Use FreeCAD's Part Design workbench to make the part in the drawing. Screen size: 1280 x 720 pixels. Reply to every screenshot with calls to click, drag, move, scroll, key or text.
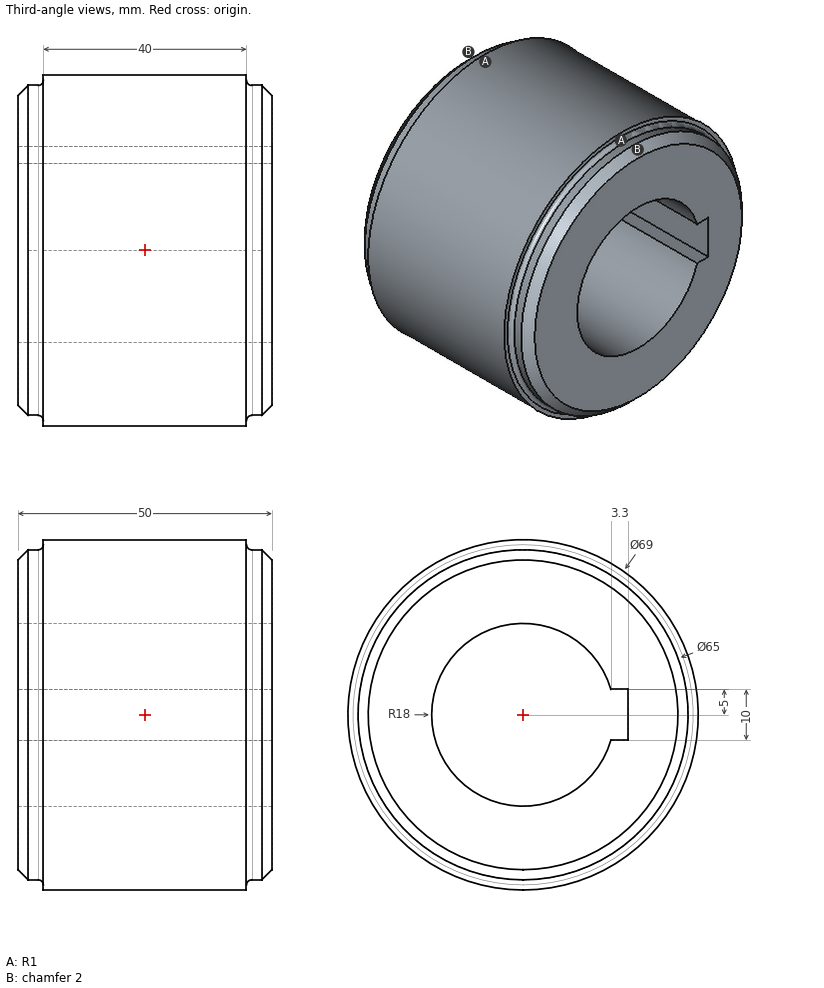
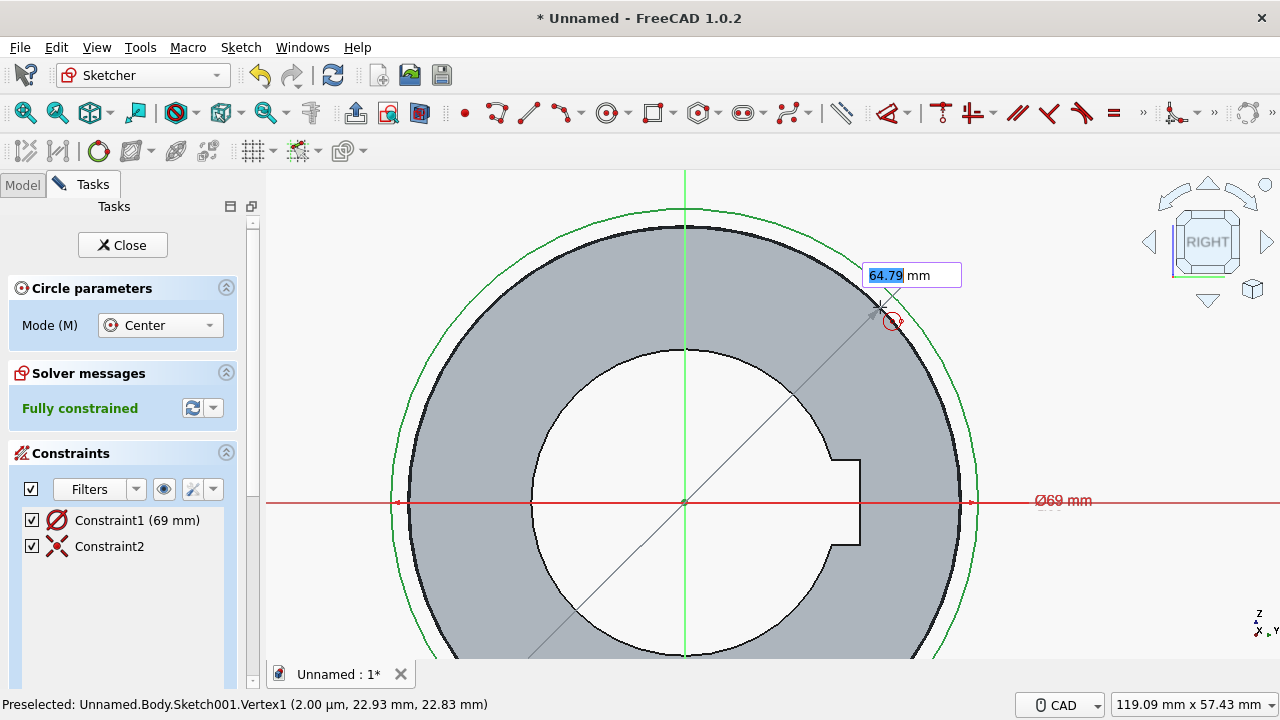
text(65)
key(Return)
key(Escape)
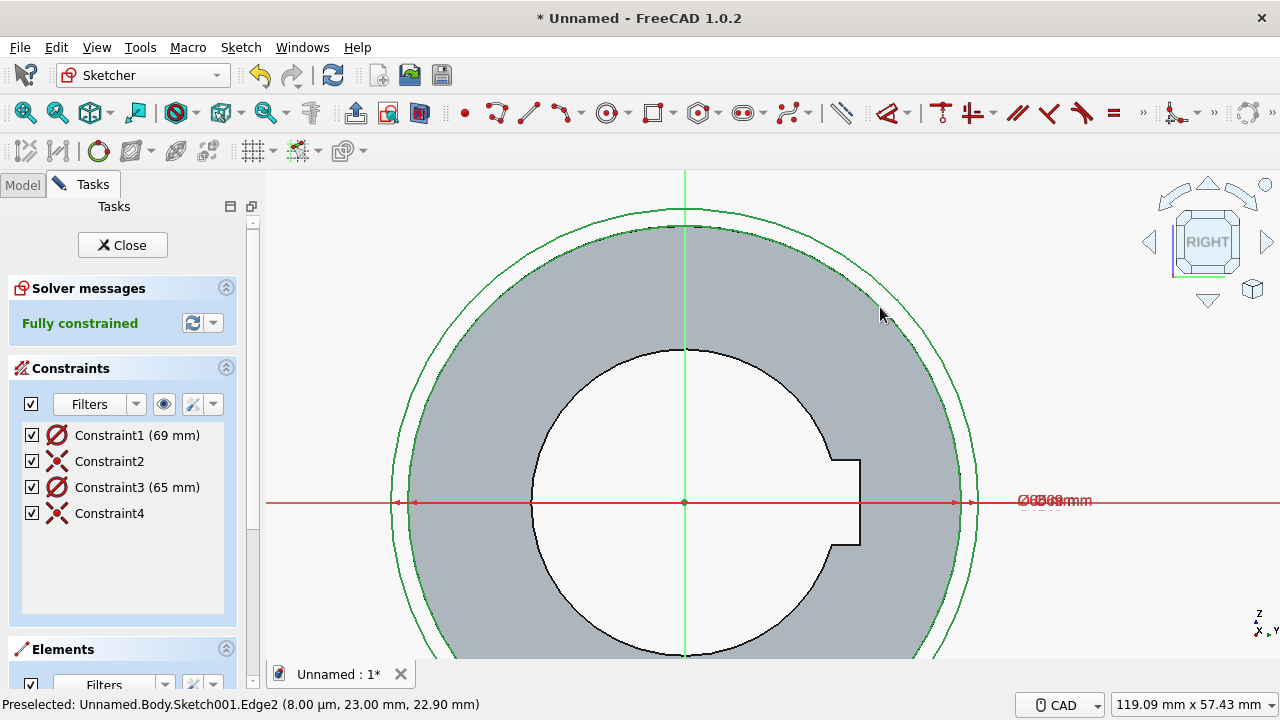
click(123, 245)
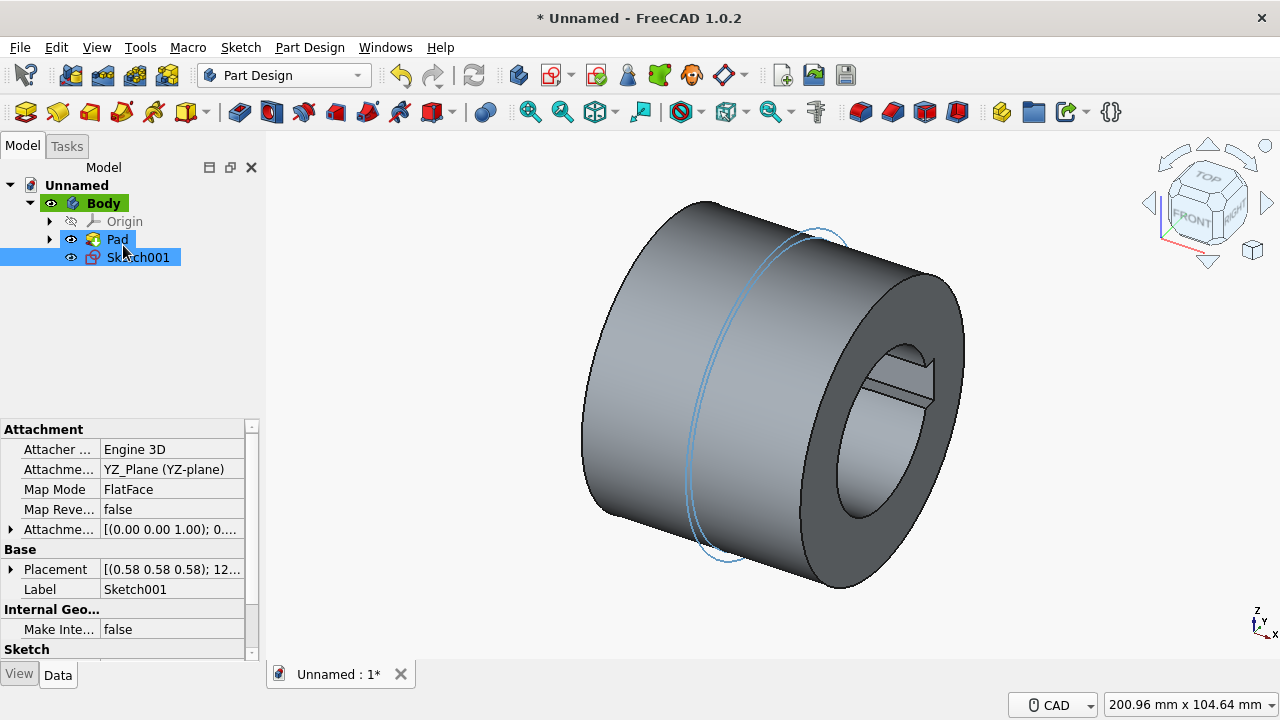
click(26, 112)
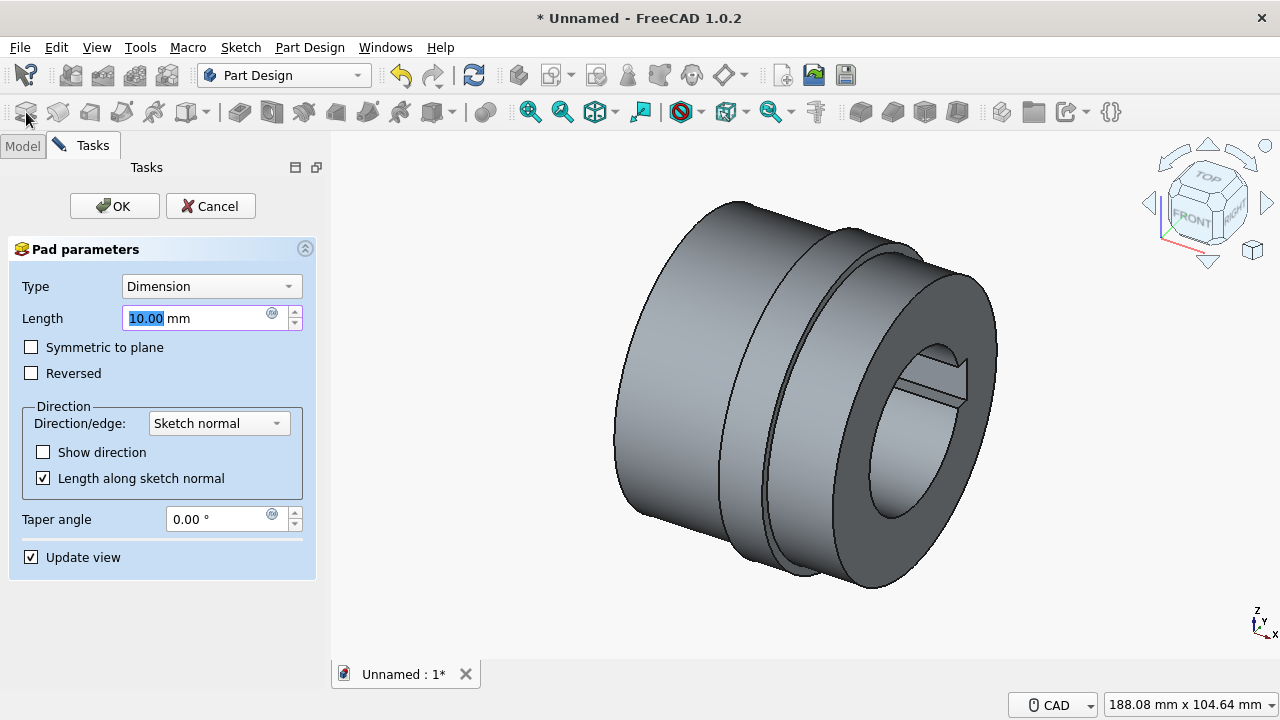
text(40)
key(Tab)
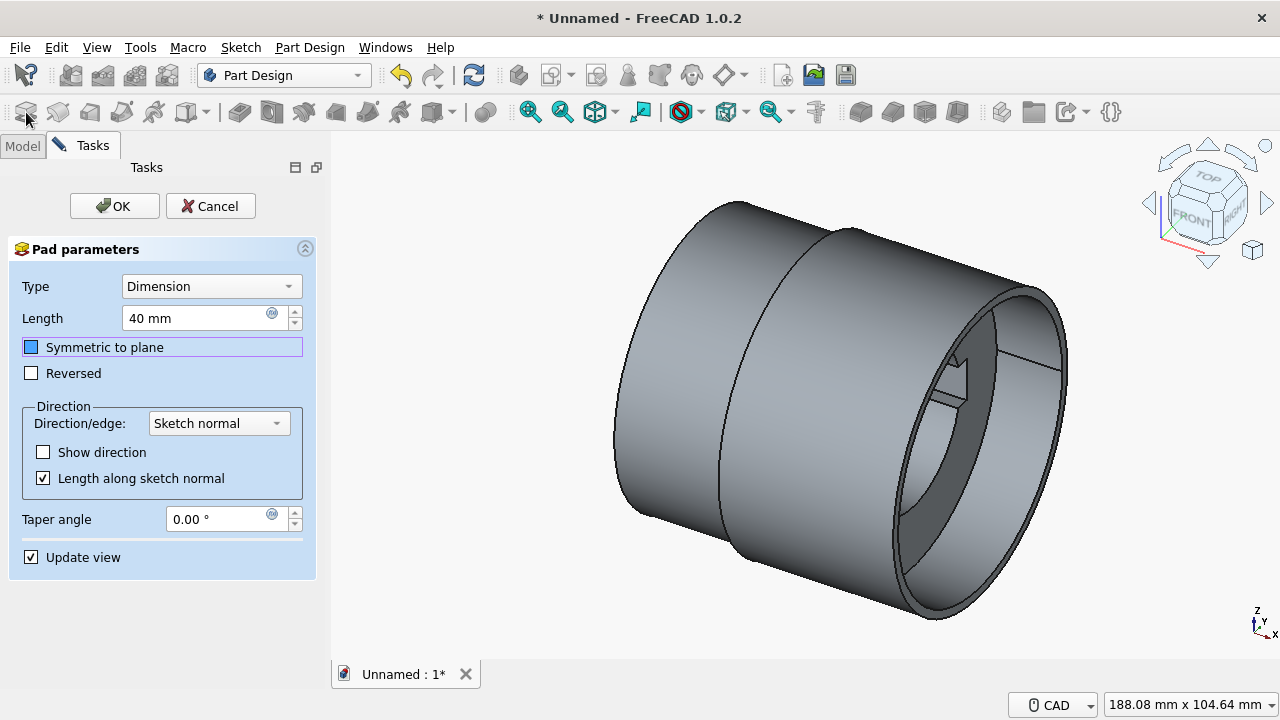
click(30, 347)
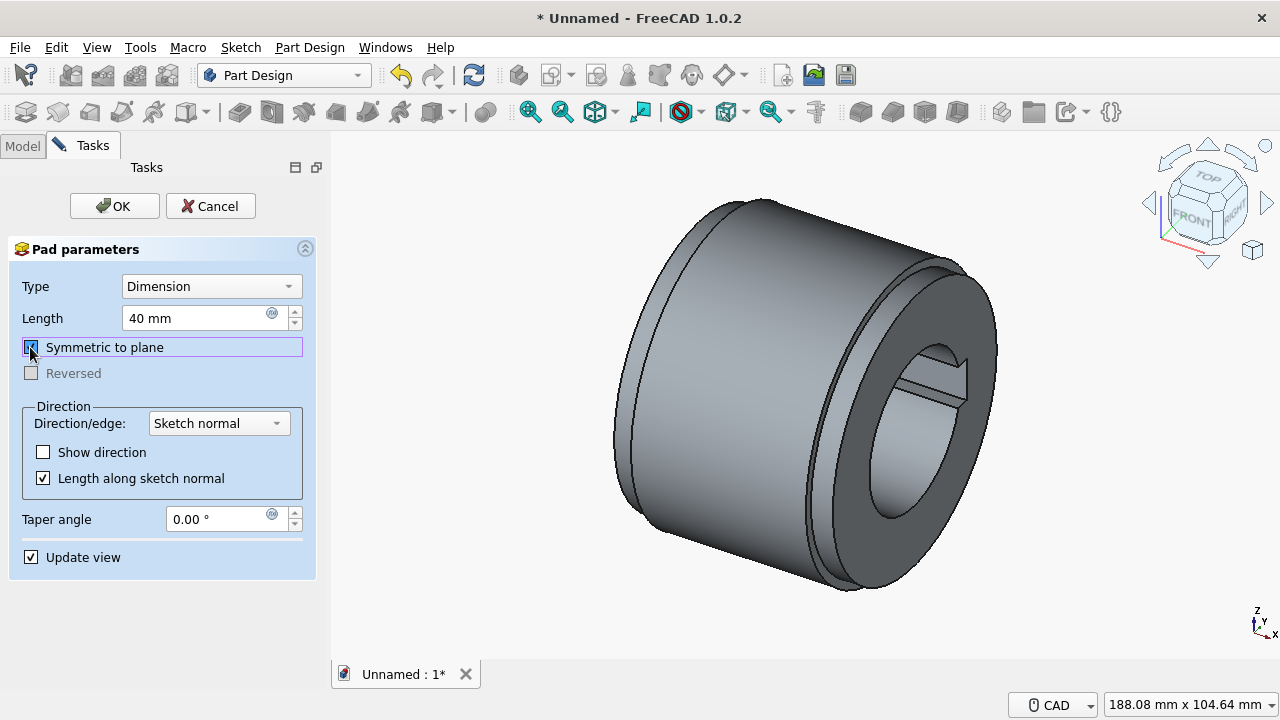
click(115, 206)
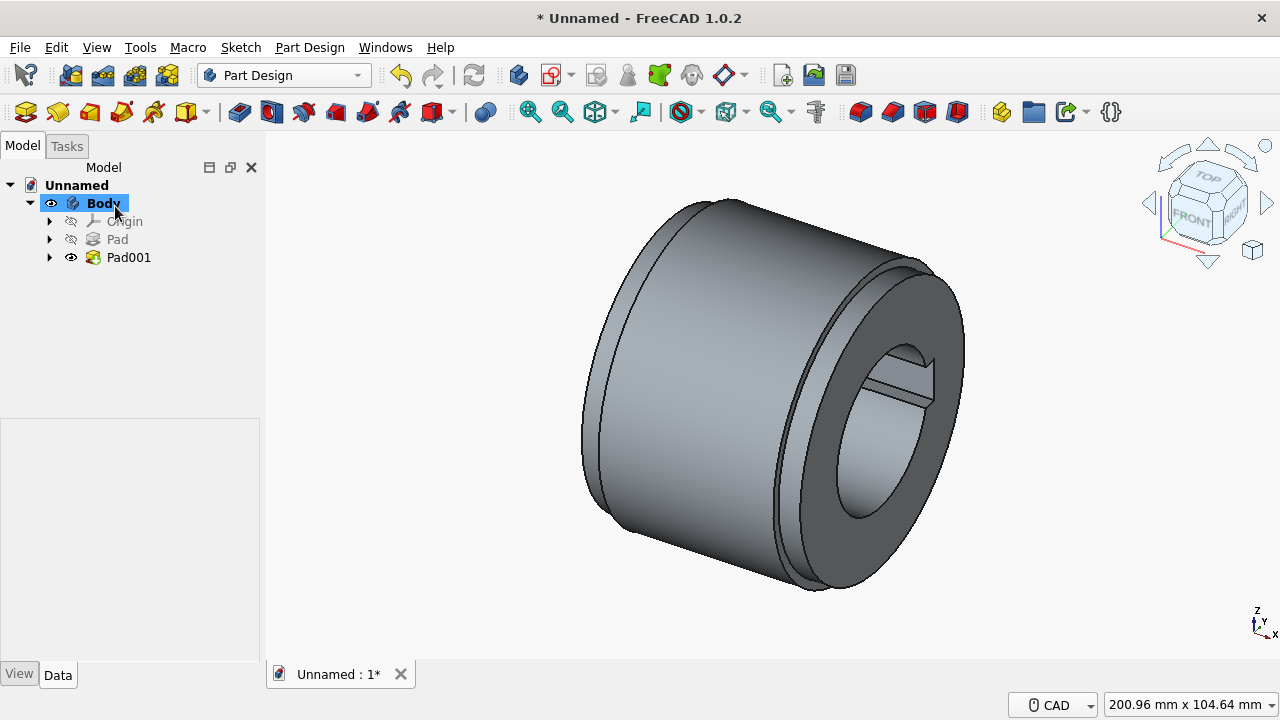
key(v)
key(f)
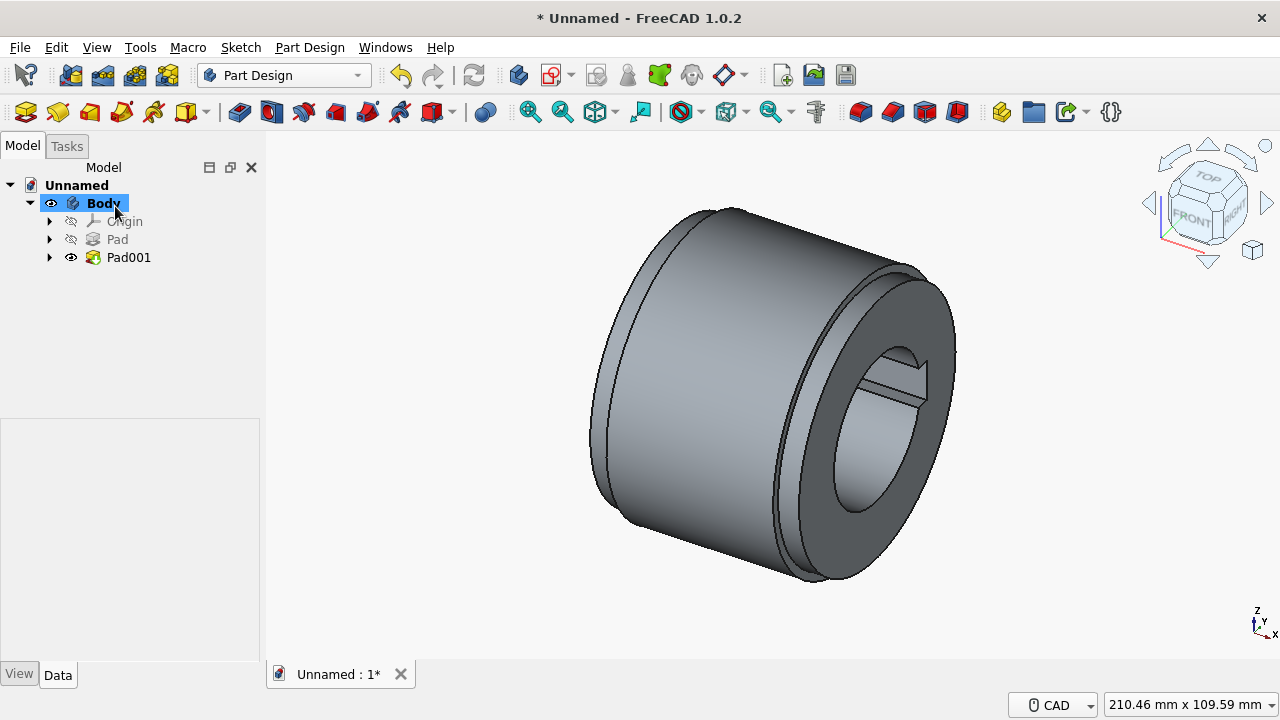
key(0)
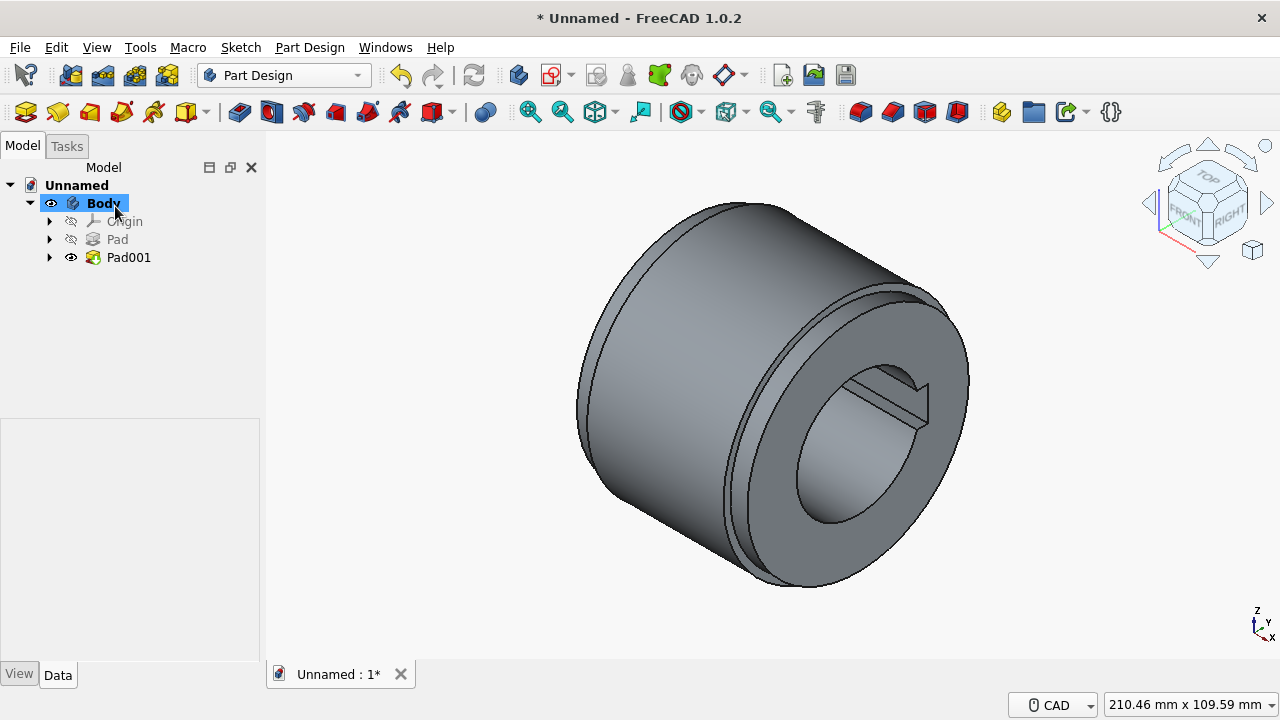
key(2)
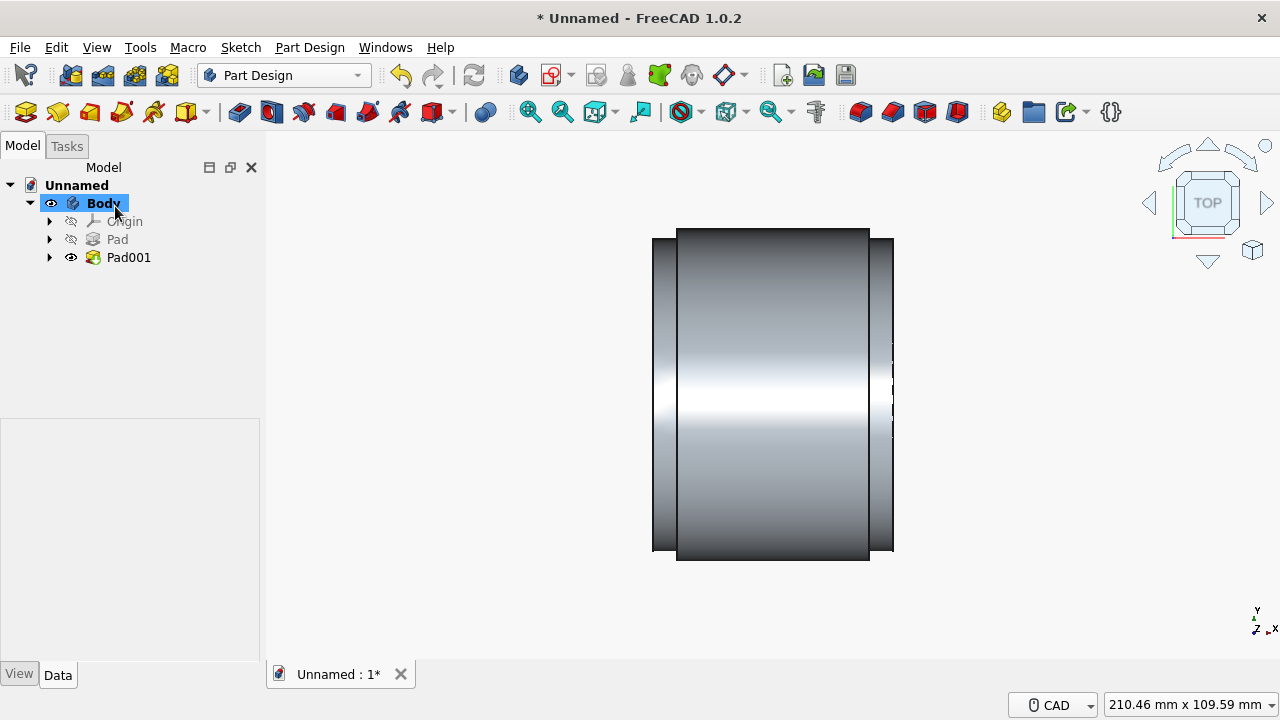
key(1)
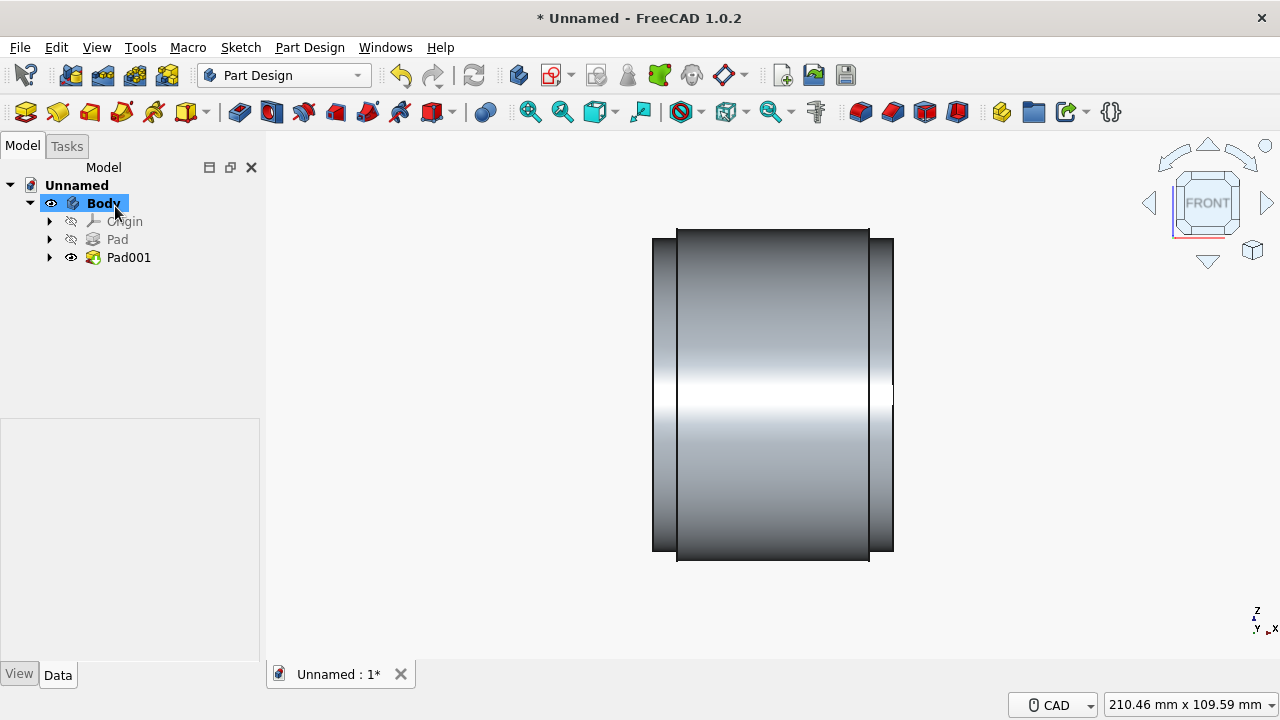
key(3)